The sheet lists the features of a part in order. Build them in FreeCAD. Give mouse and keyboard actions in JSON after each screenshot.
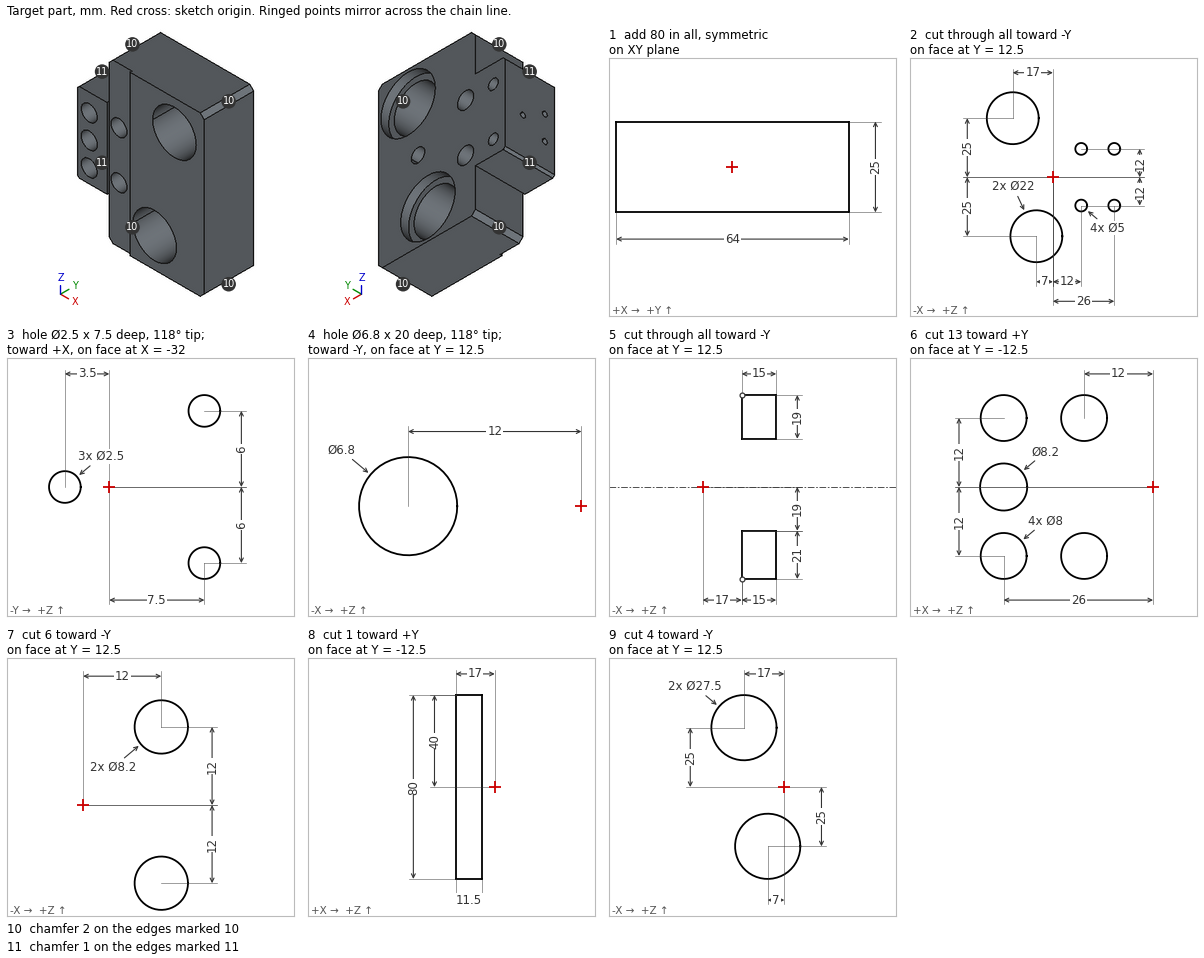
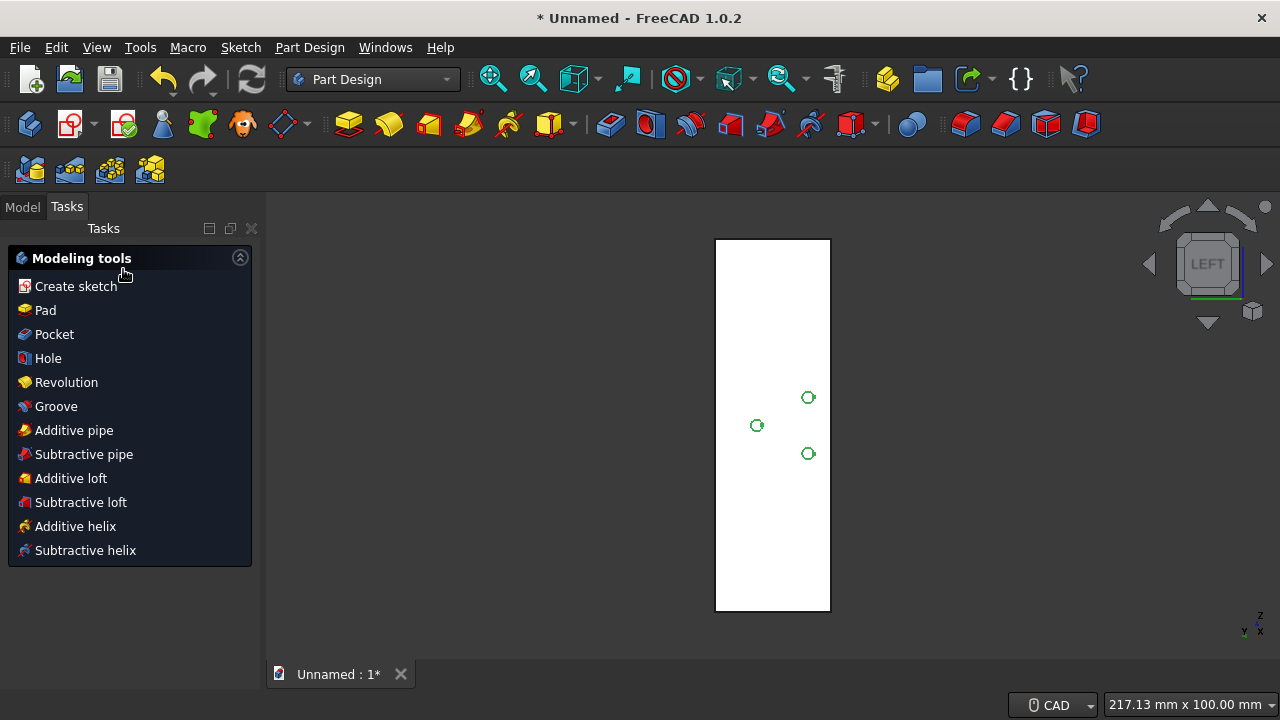
{"action": "left_click", "coordinate": [652, 124]}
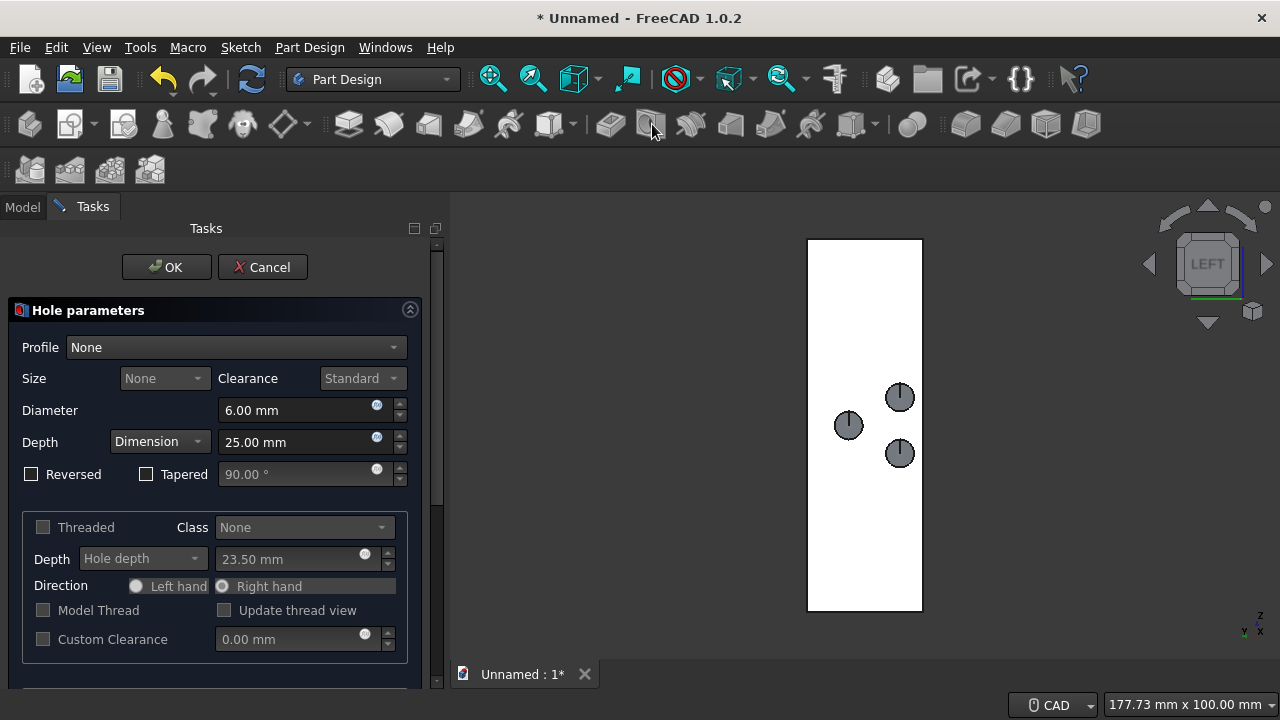
{"action": "triple_click", "coordinate": [305, 410]}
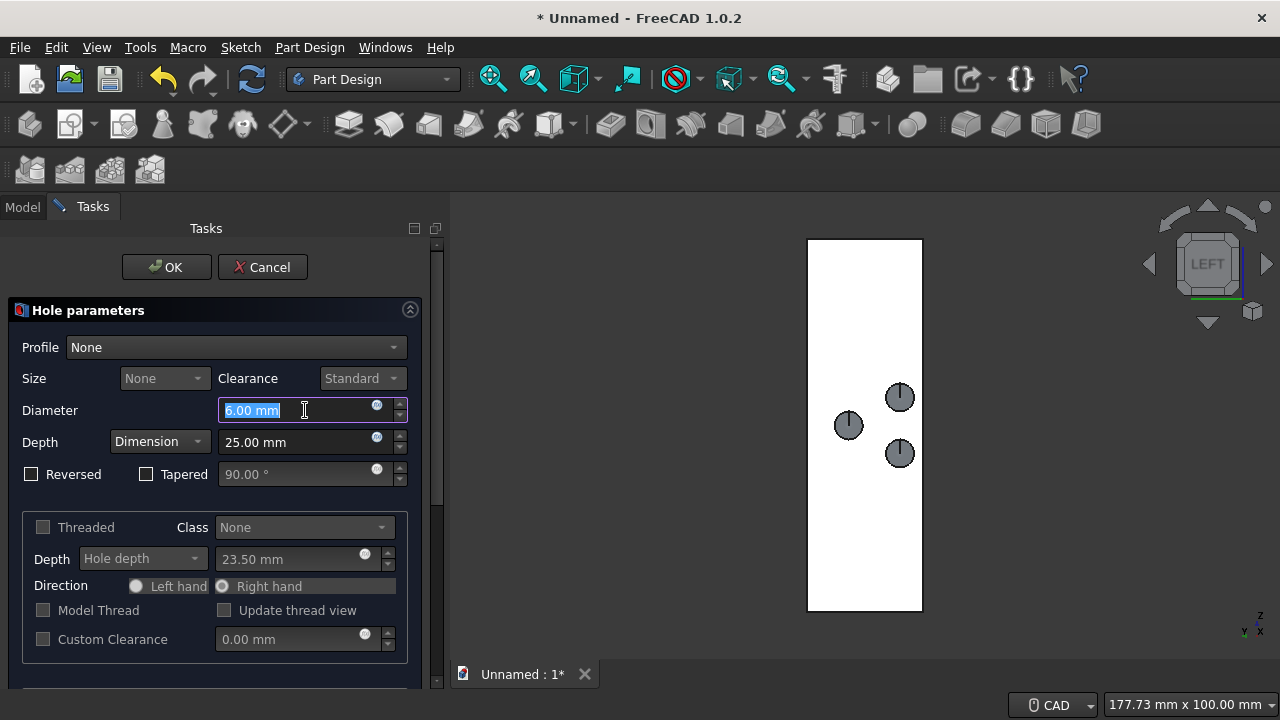
{"action": "type", "text": "2.5"}
{"action": "key", "text": "Tab"}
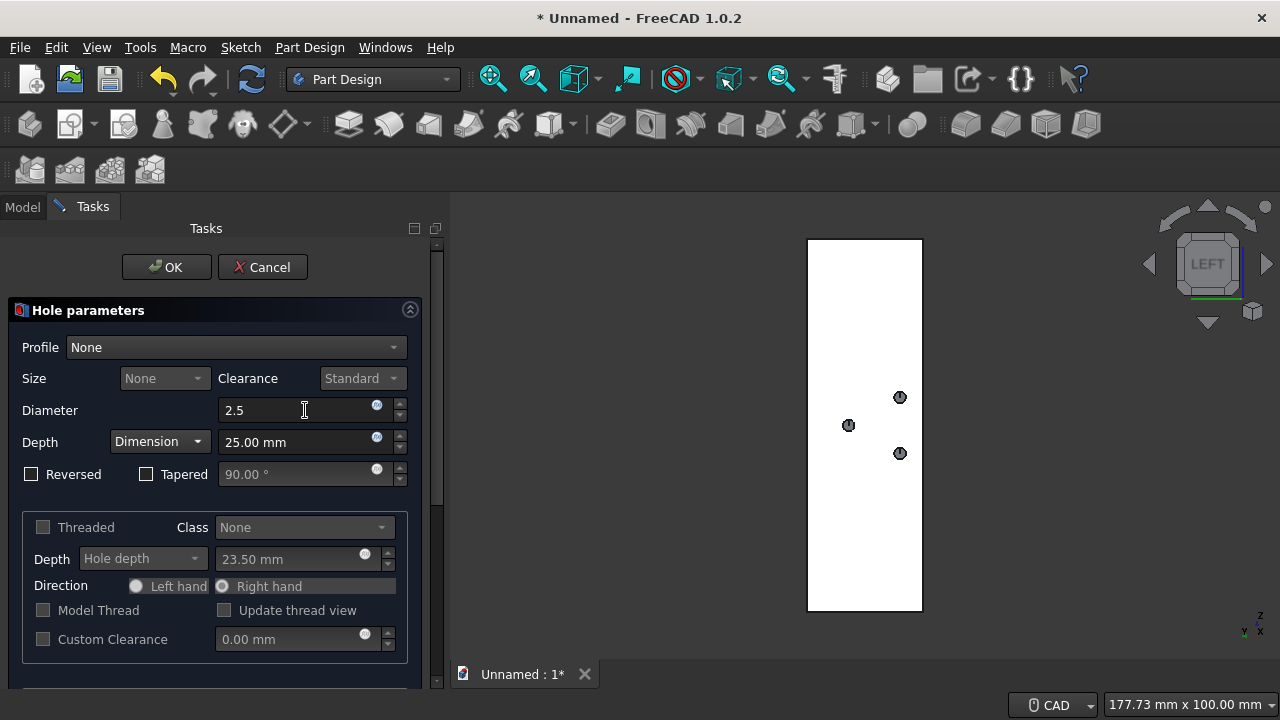
{"action": "triple_click", "coordinate": [305, 442]}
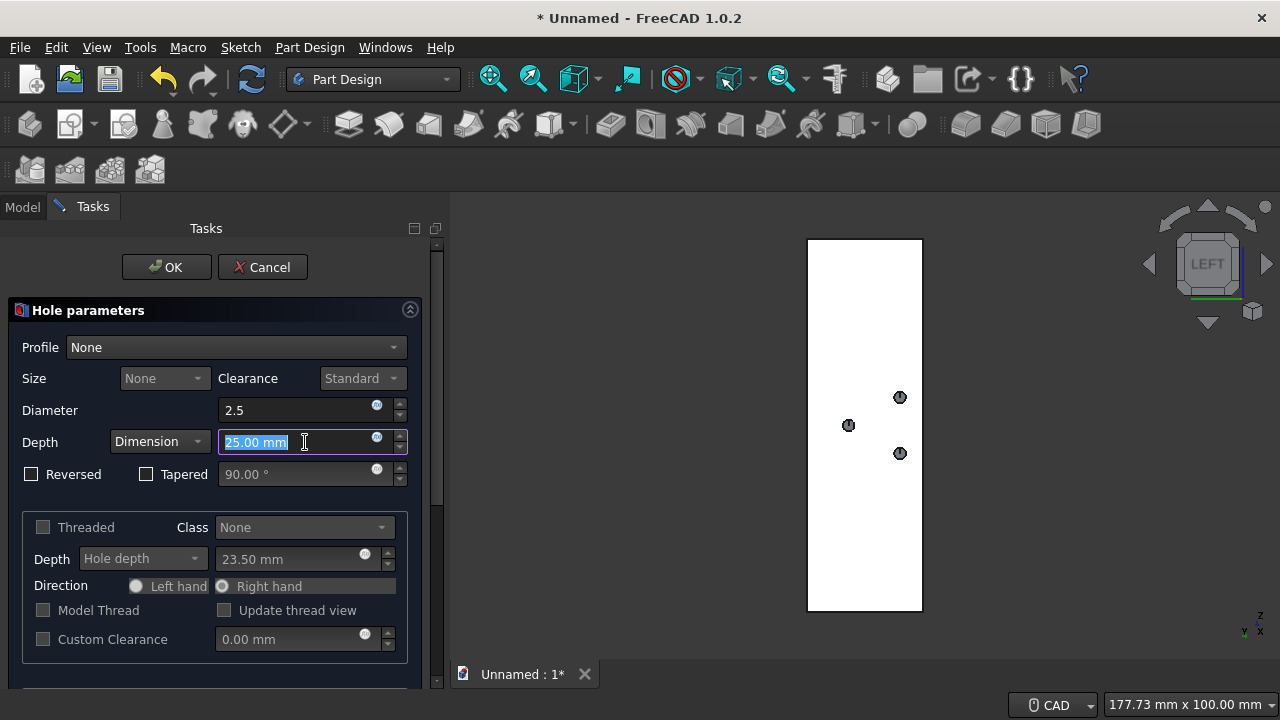
{"action": "type", "text": "7.5"}
{"action": "key", "text": "Tab"}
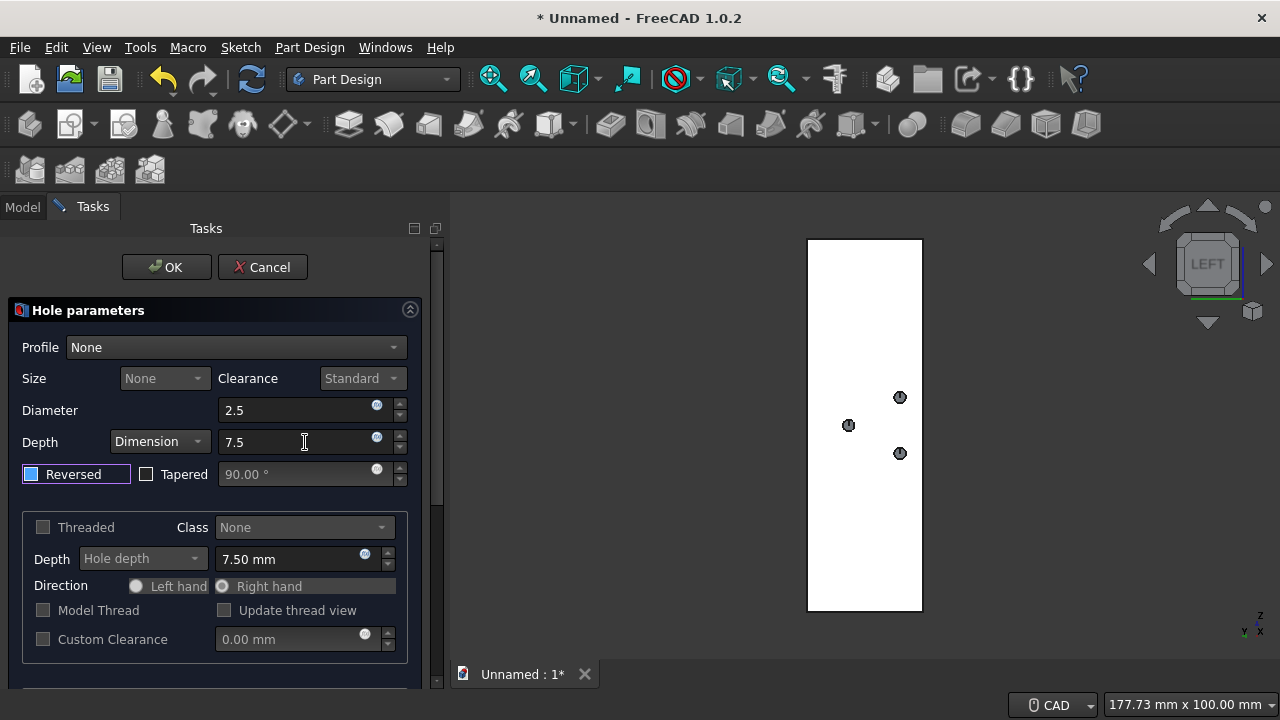
{"action": "left_click", "coordinate": [167, 267]}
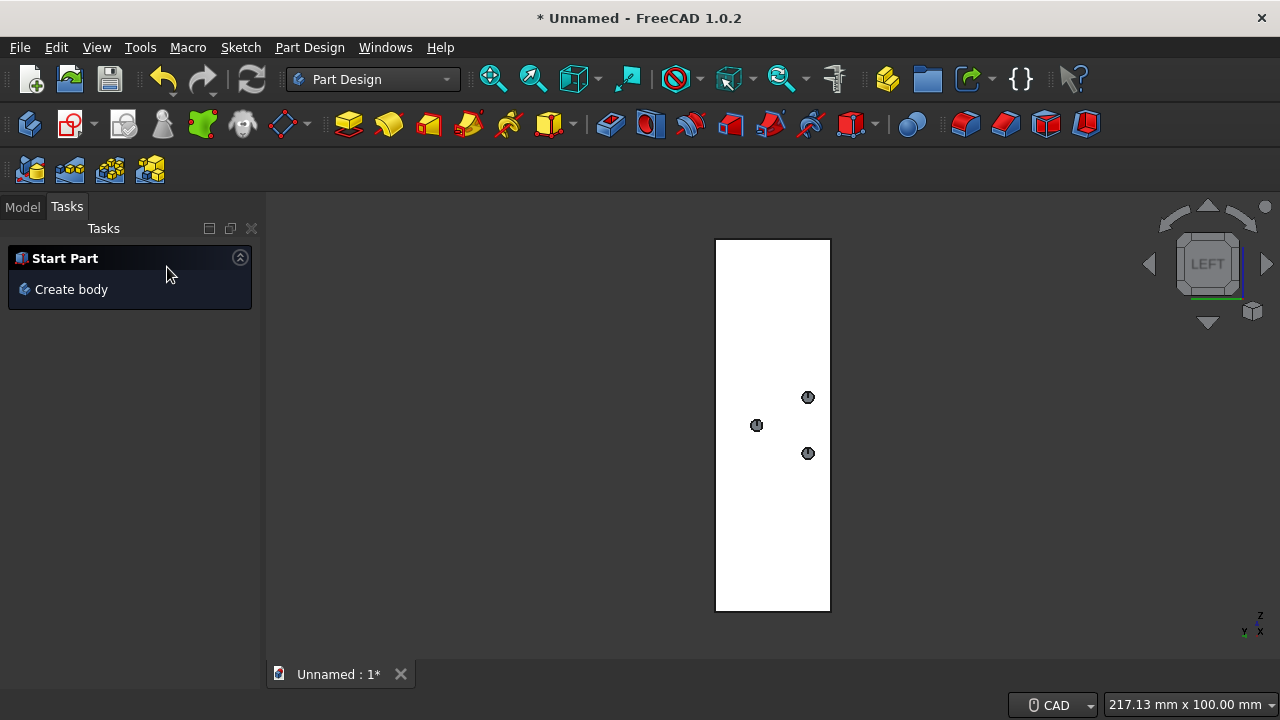
{"action": "key", "text": "4"}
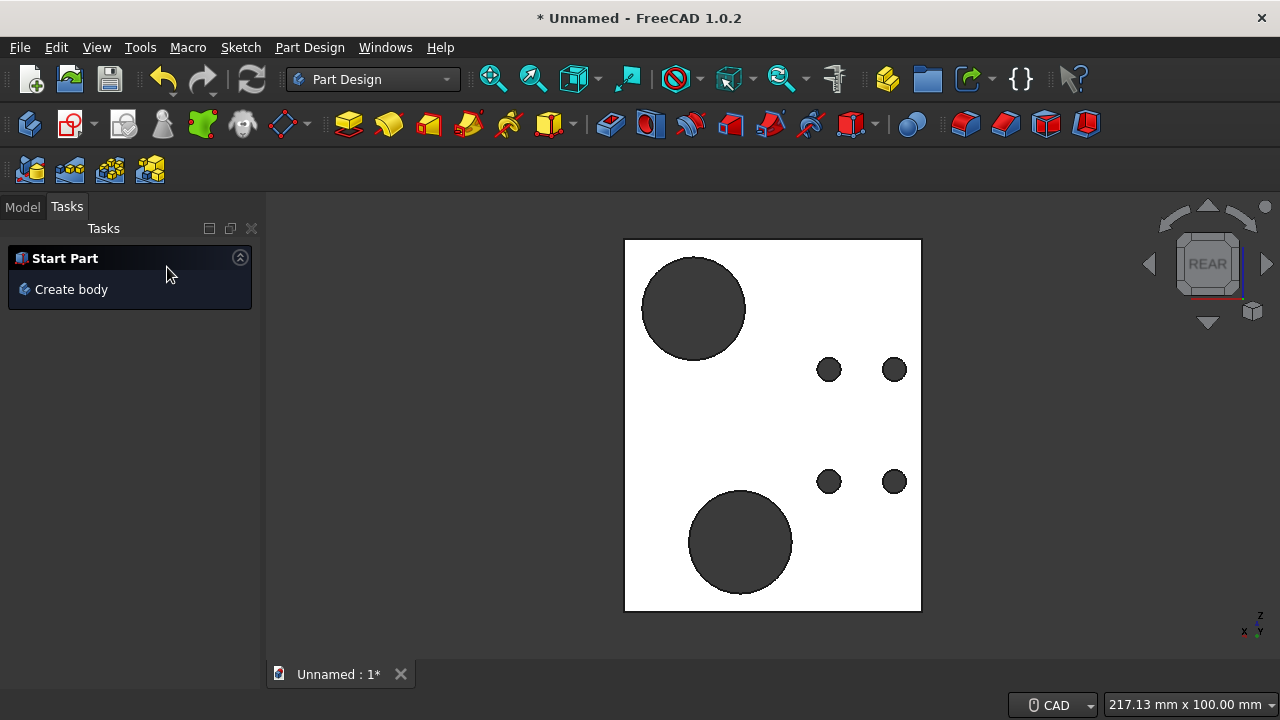
{"action": "left_click", "coordinate": [773, 425]}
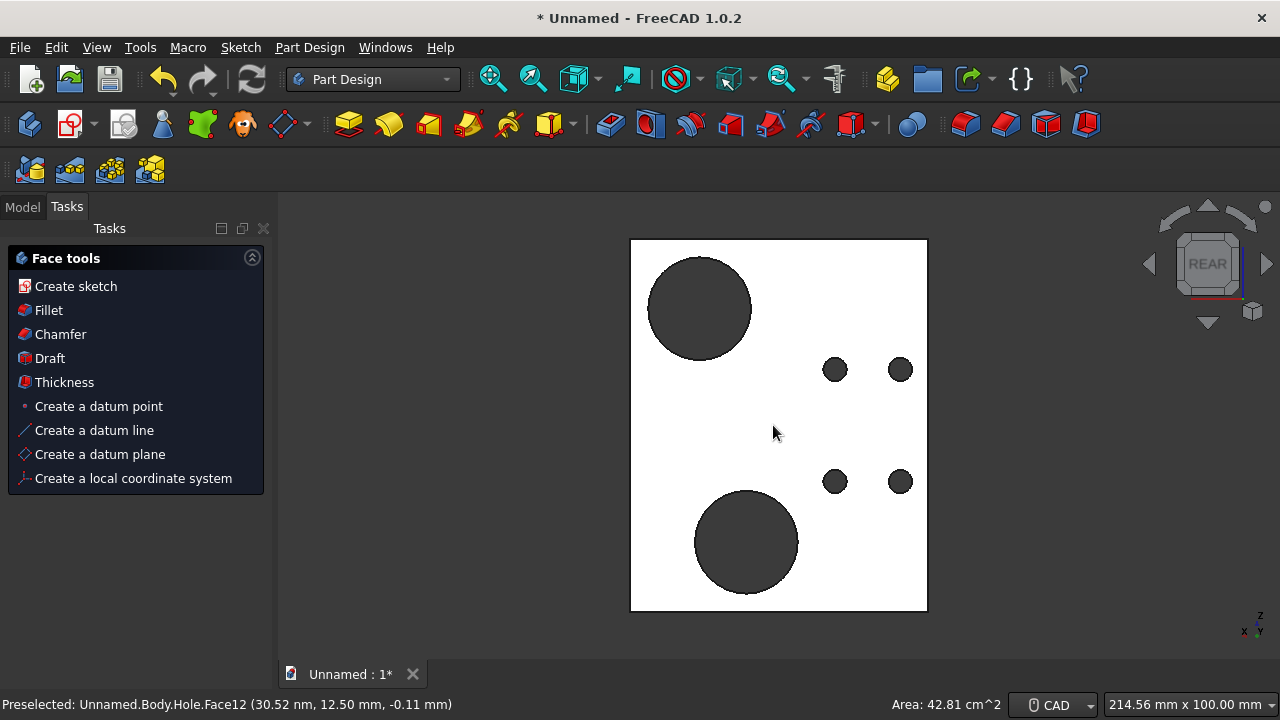
{"action": "left_click", "coordinate": [70, 124]}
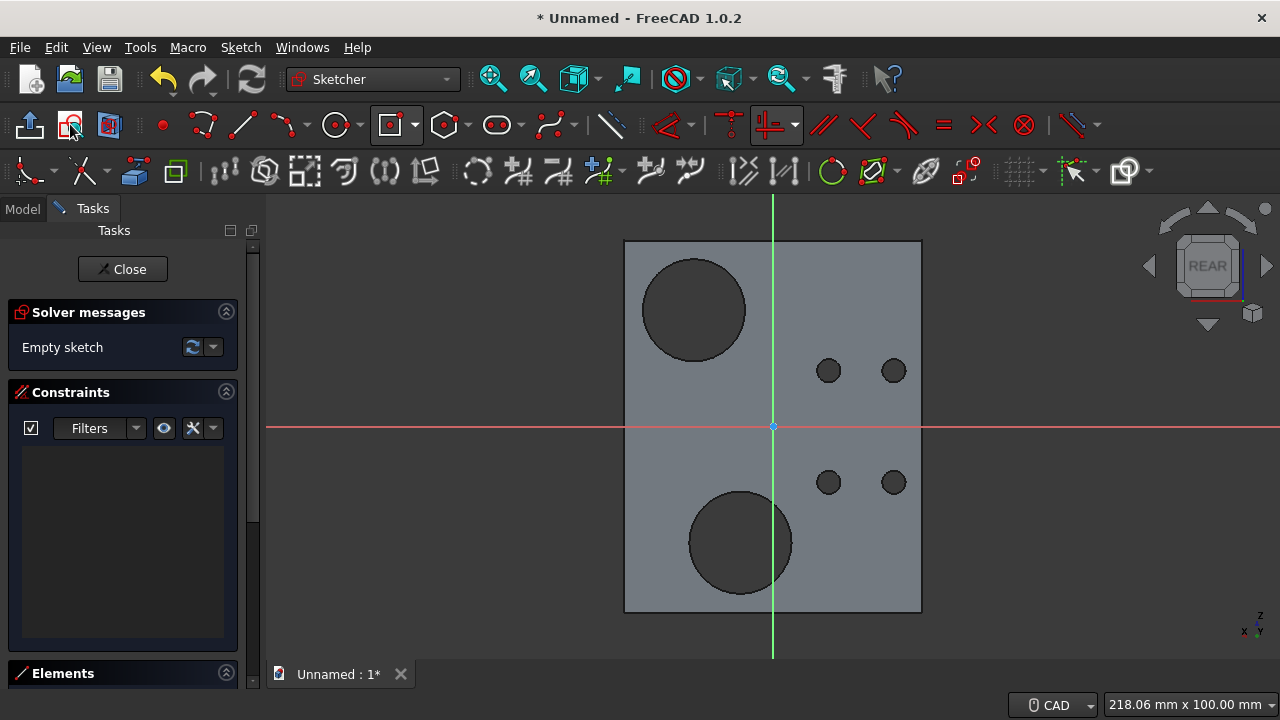
{"action": "scroll", "coordinate": [742, 427], "scroll_direction": "up", "scroll_amount": 10}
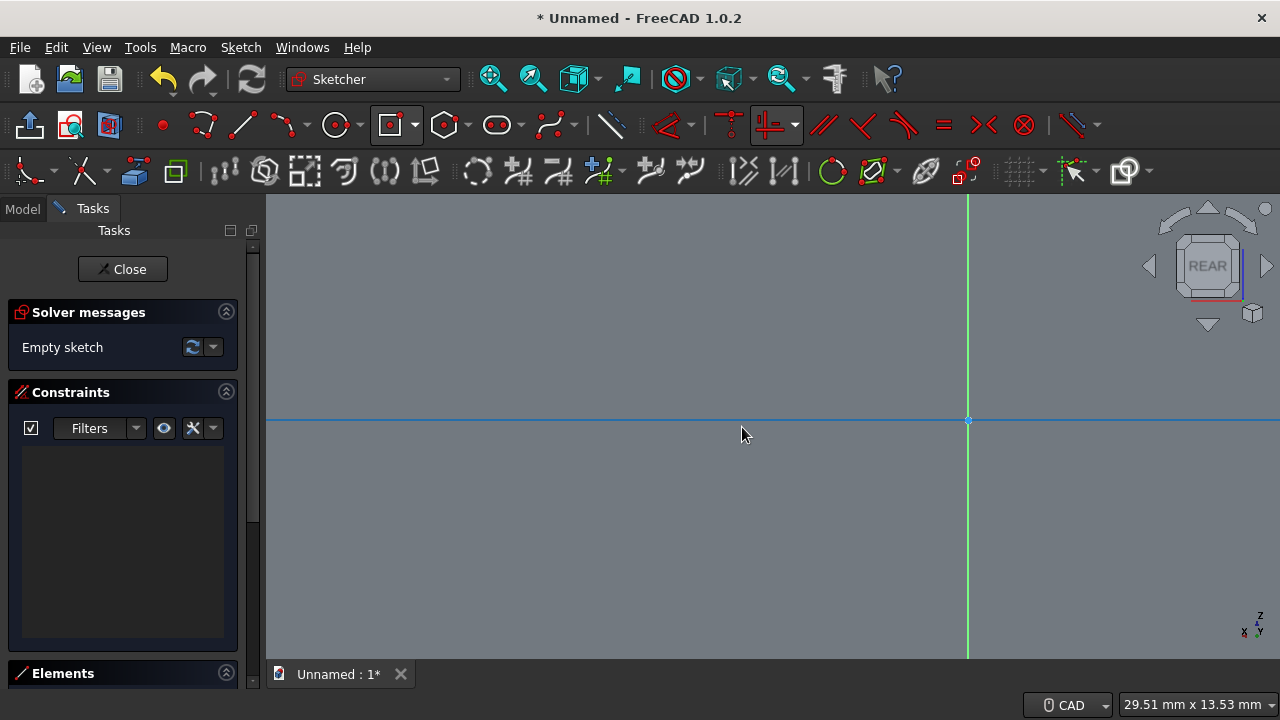
{"action": "left_click", "coordinate": [336, 126]}